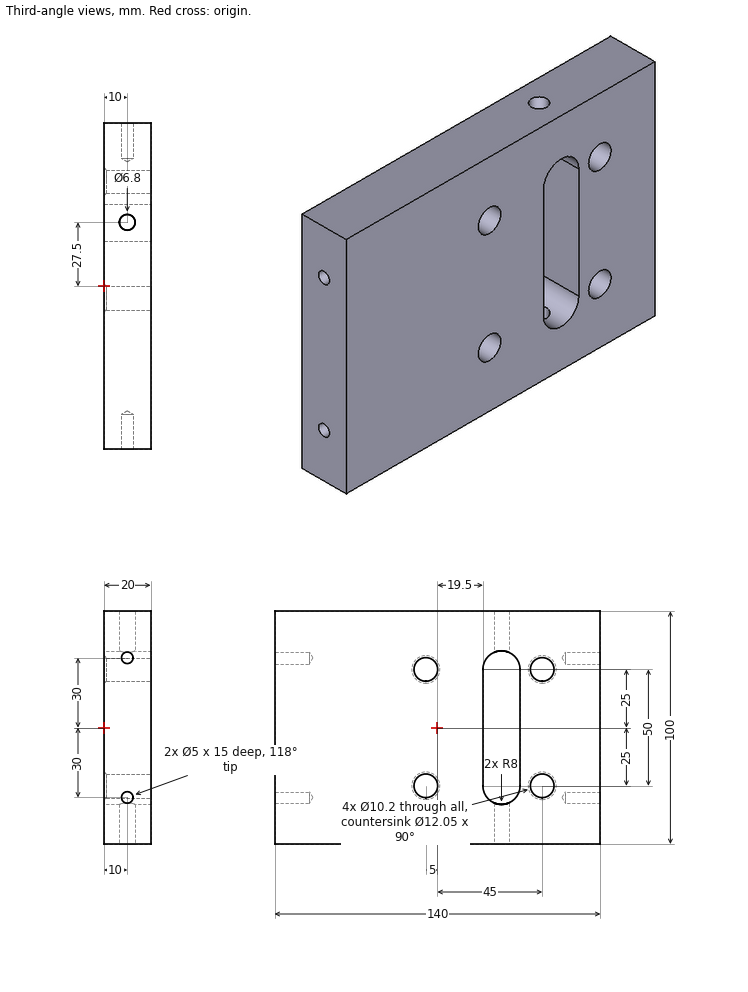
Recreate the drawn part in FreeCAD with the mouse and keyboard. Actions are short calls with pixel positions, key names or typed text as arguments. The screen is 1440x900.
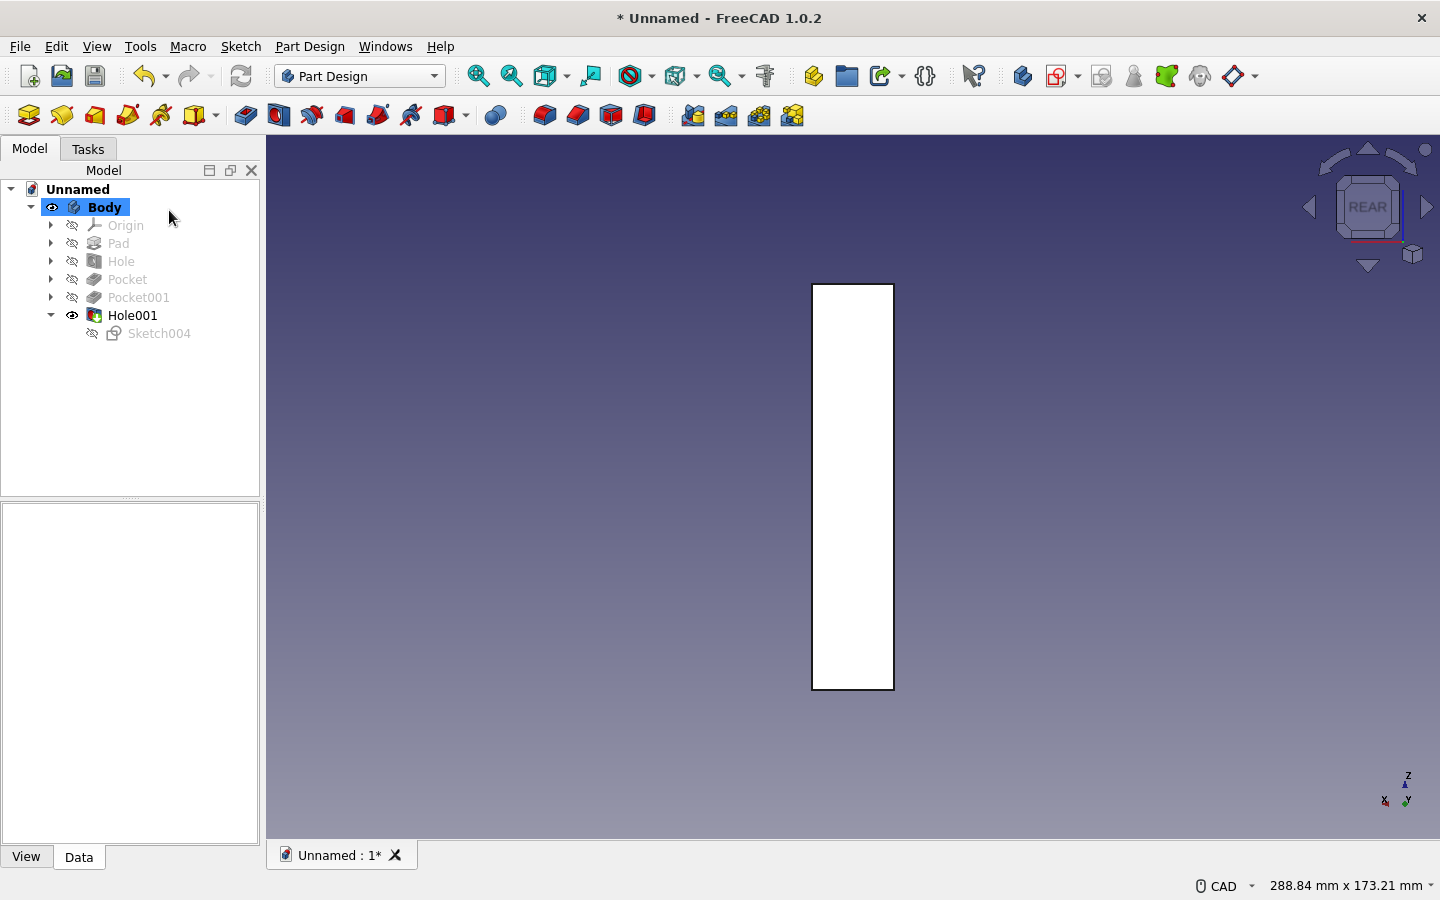
click(853, 486)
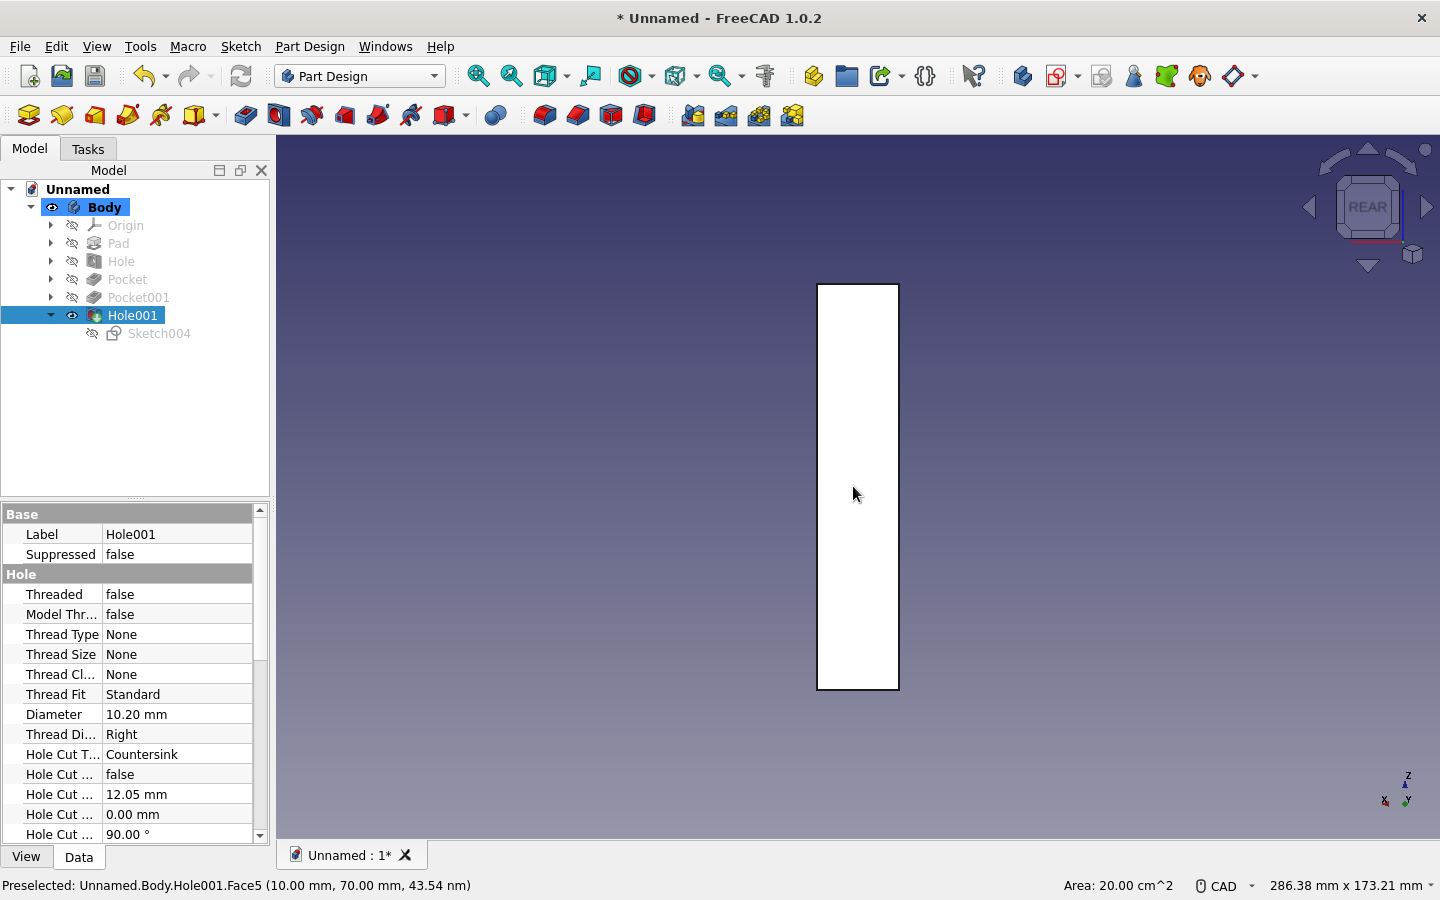
click(1056, 76)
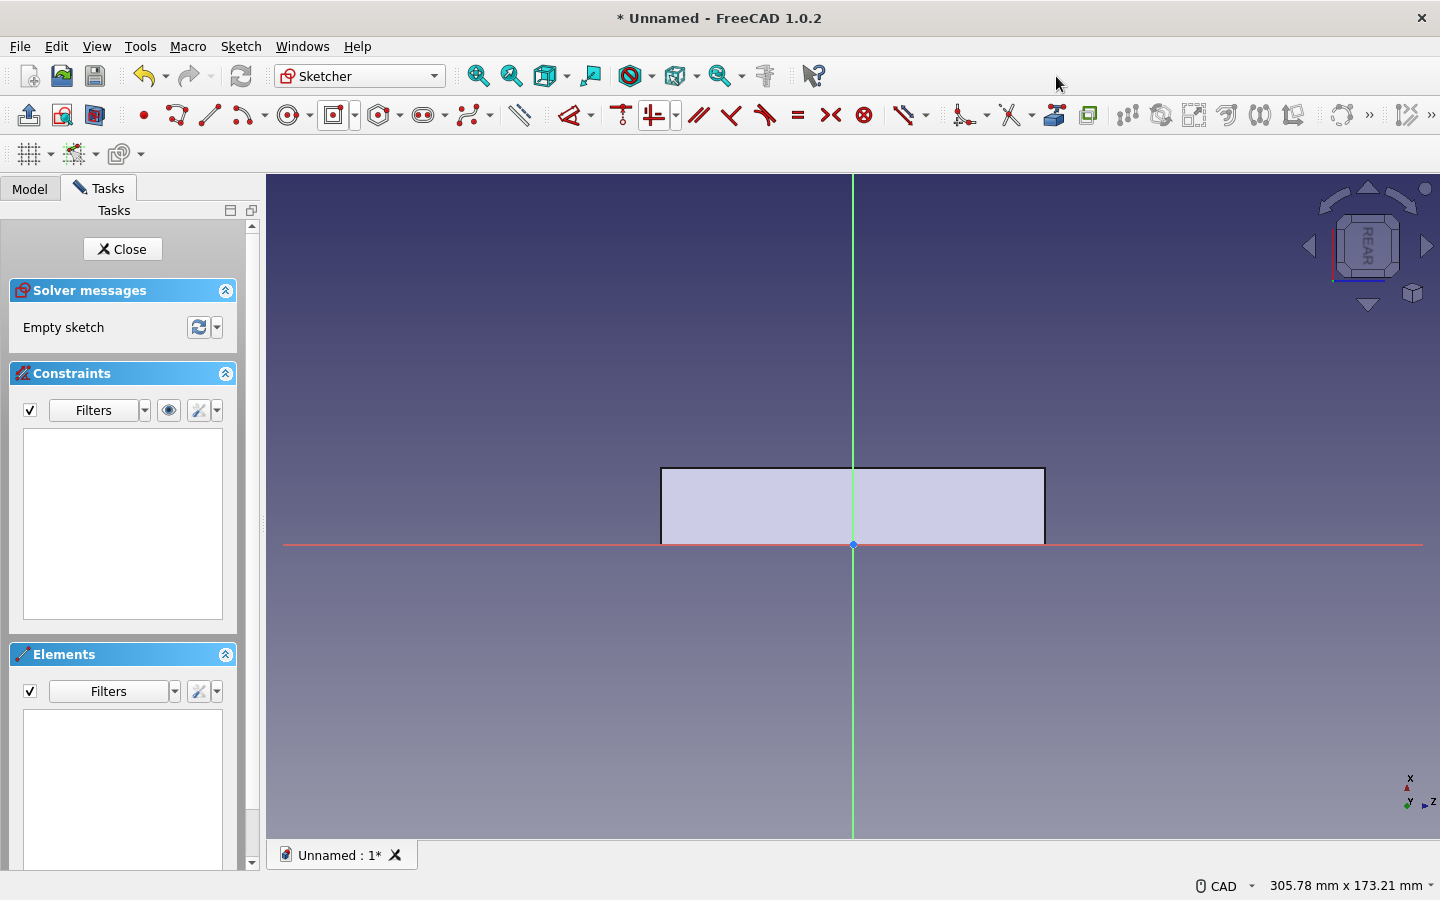
scroll(893, 529, up, 5)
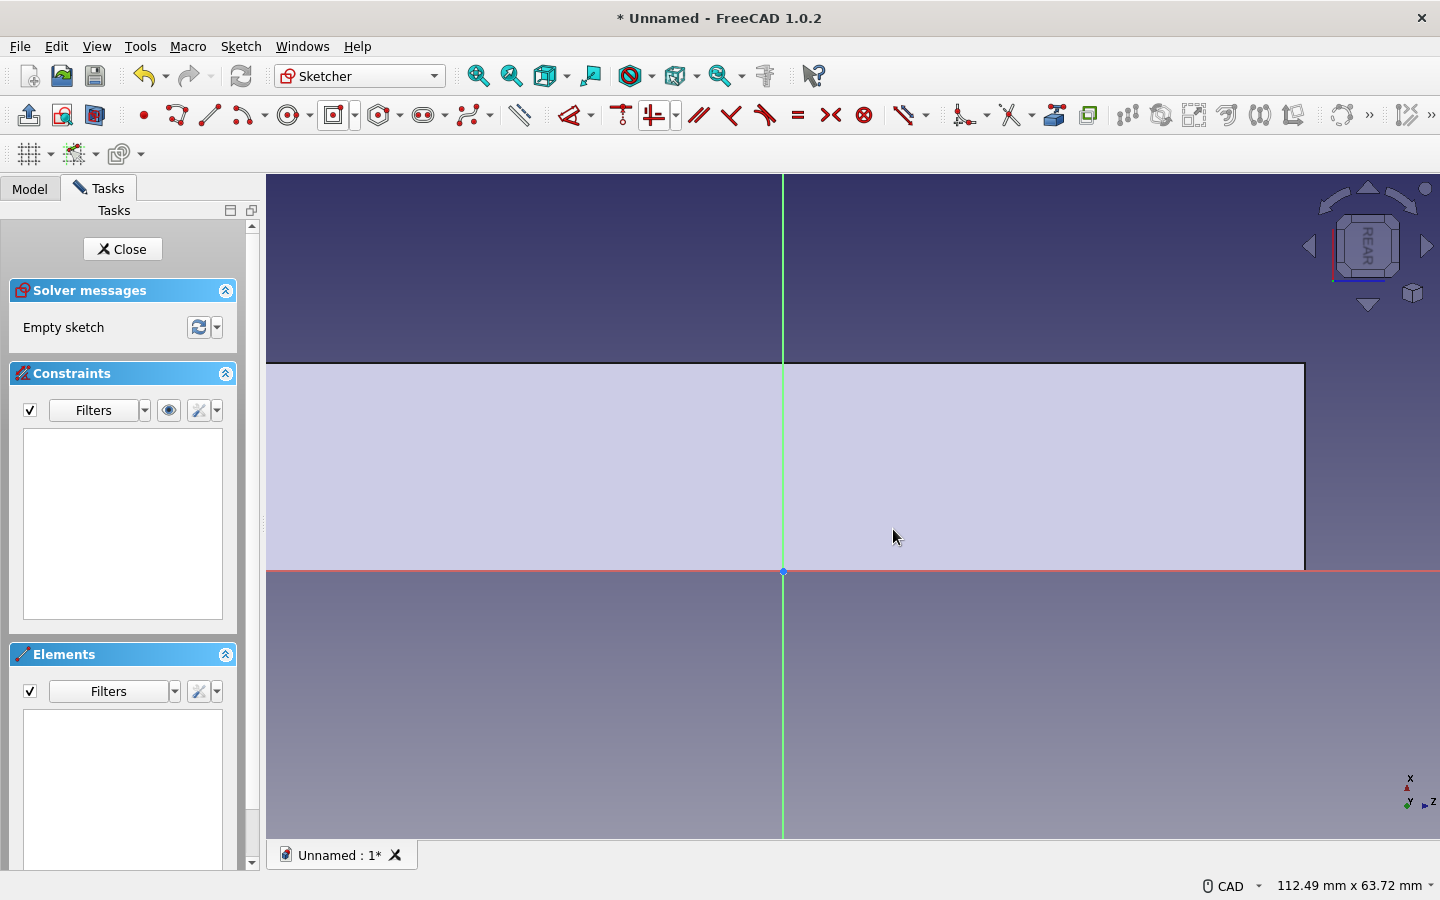
click(288, 116)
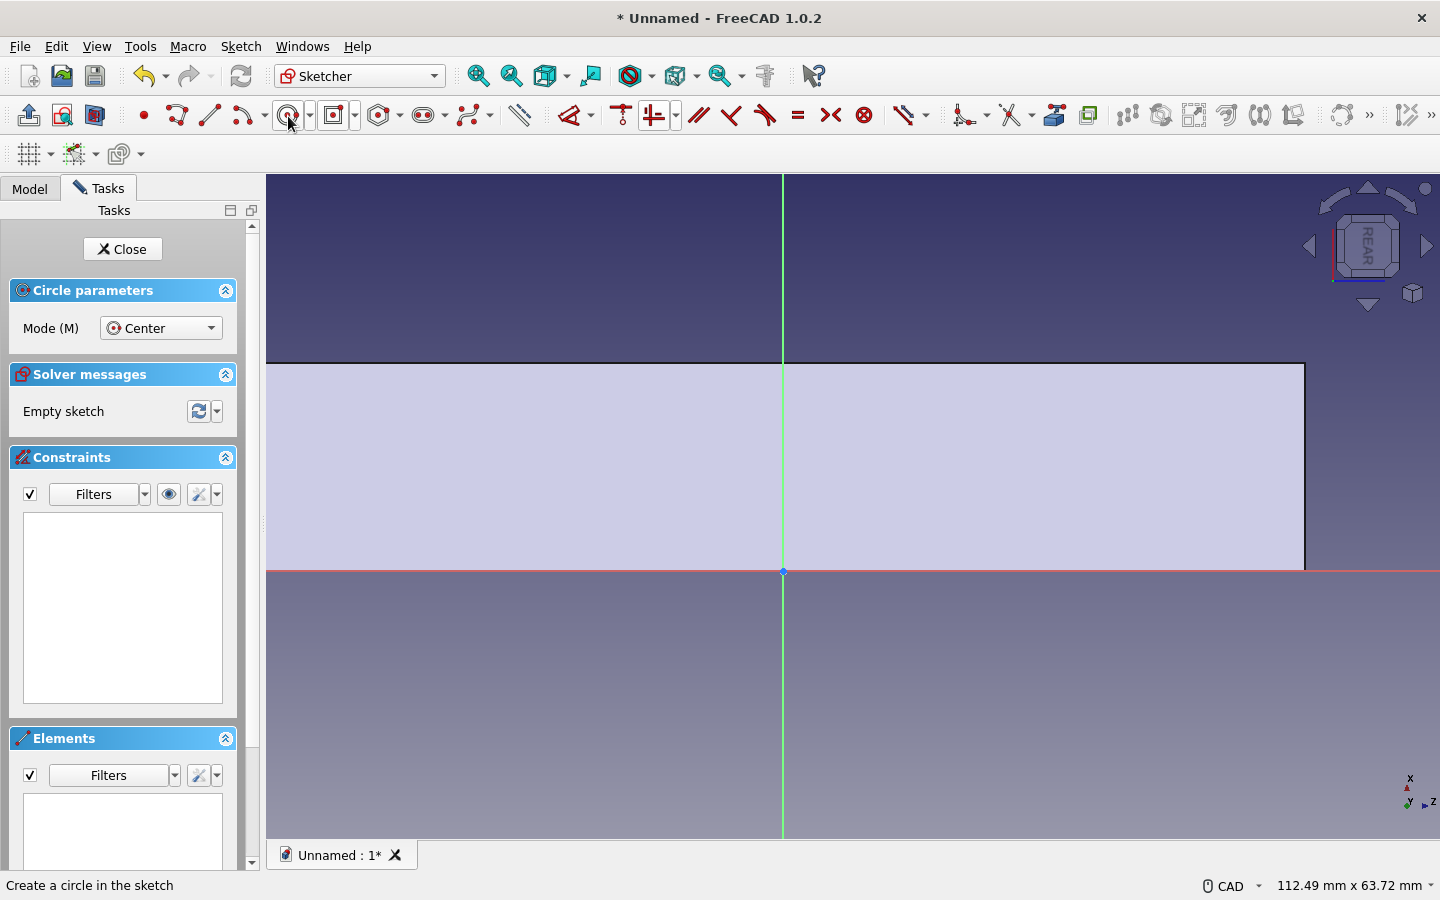
click(470, 467)
move(489, 448)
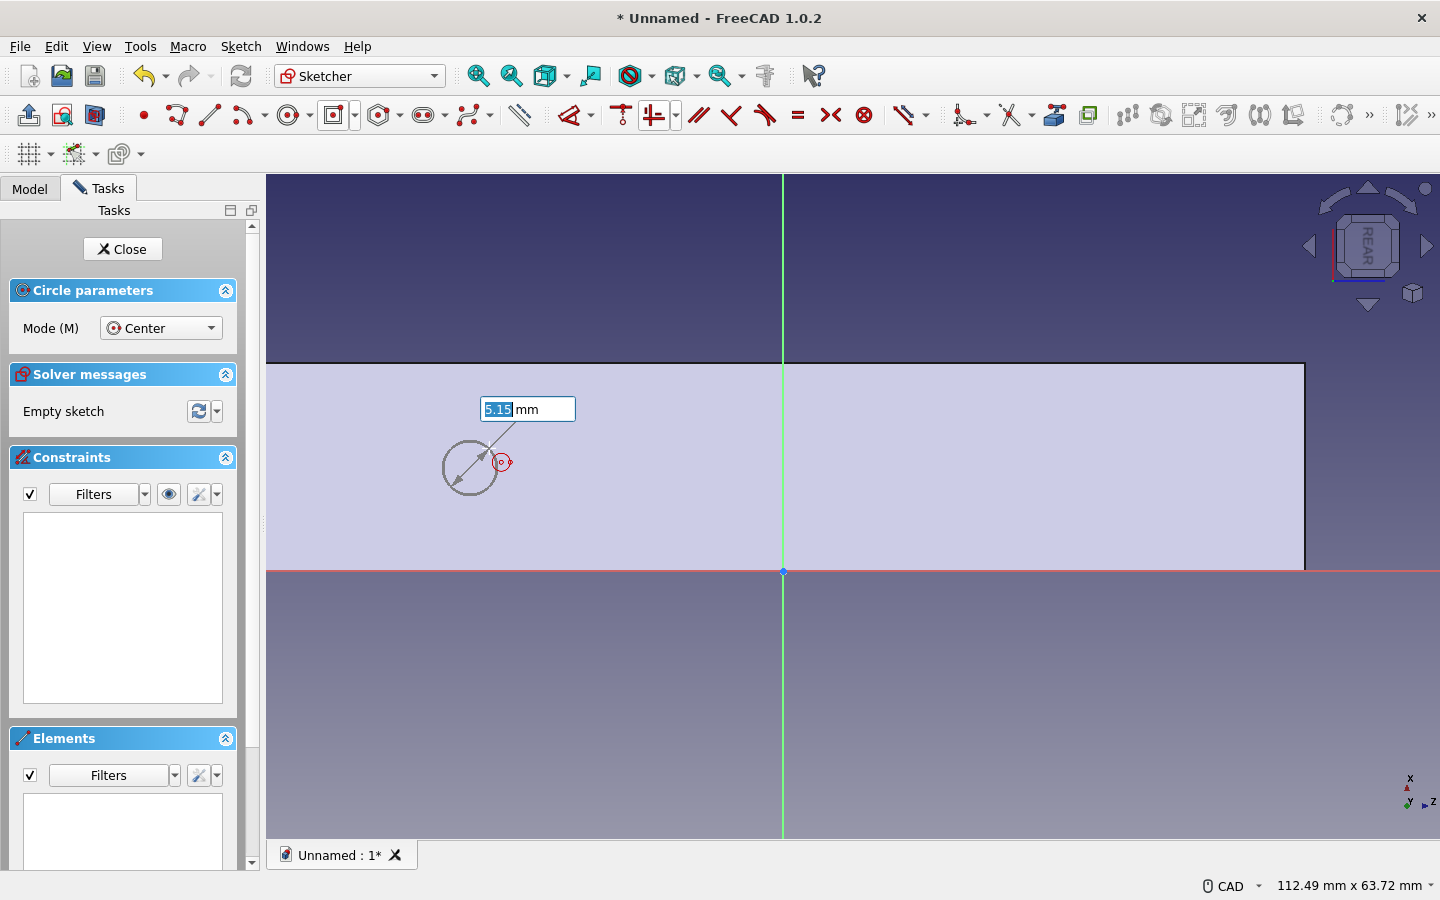
text(5)
key(Return)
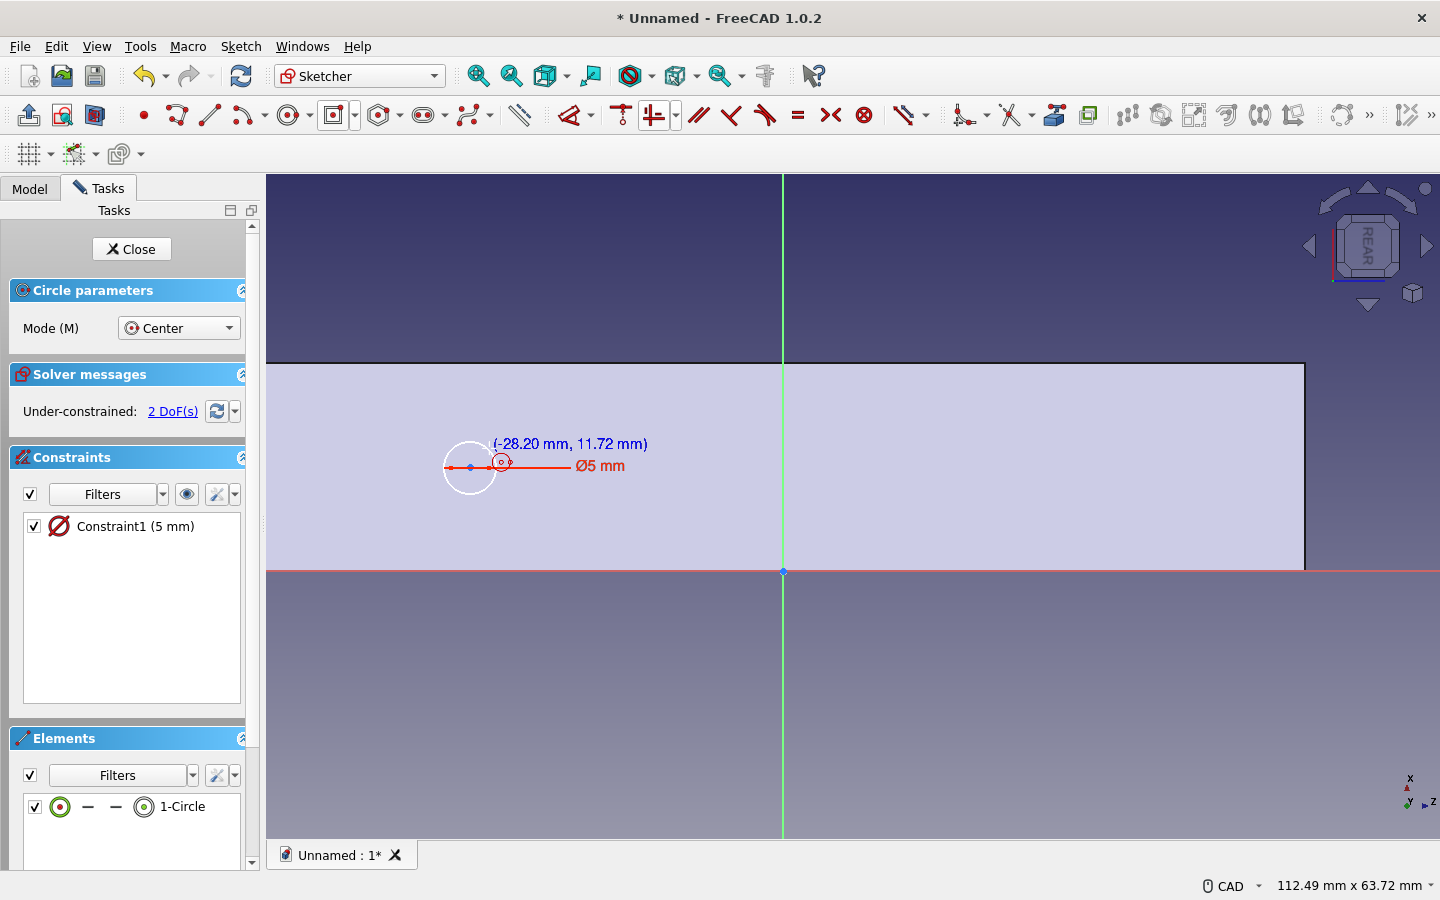
click(1096, 467)
move(1115, 448)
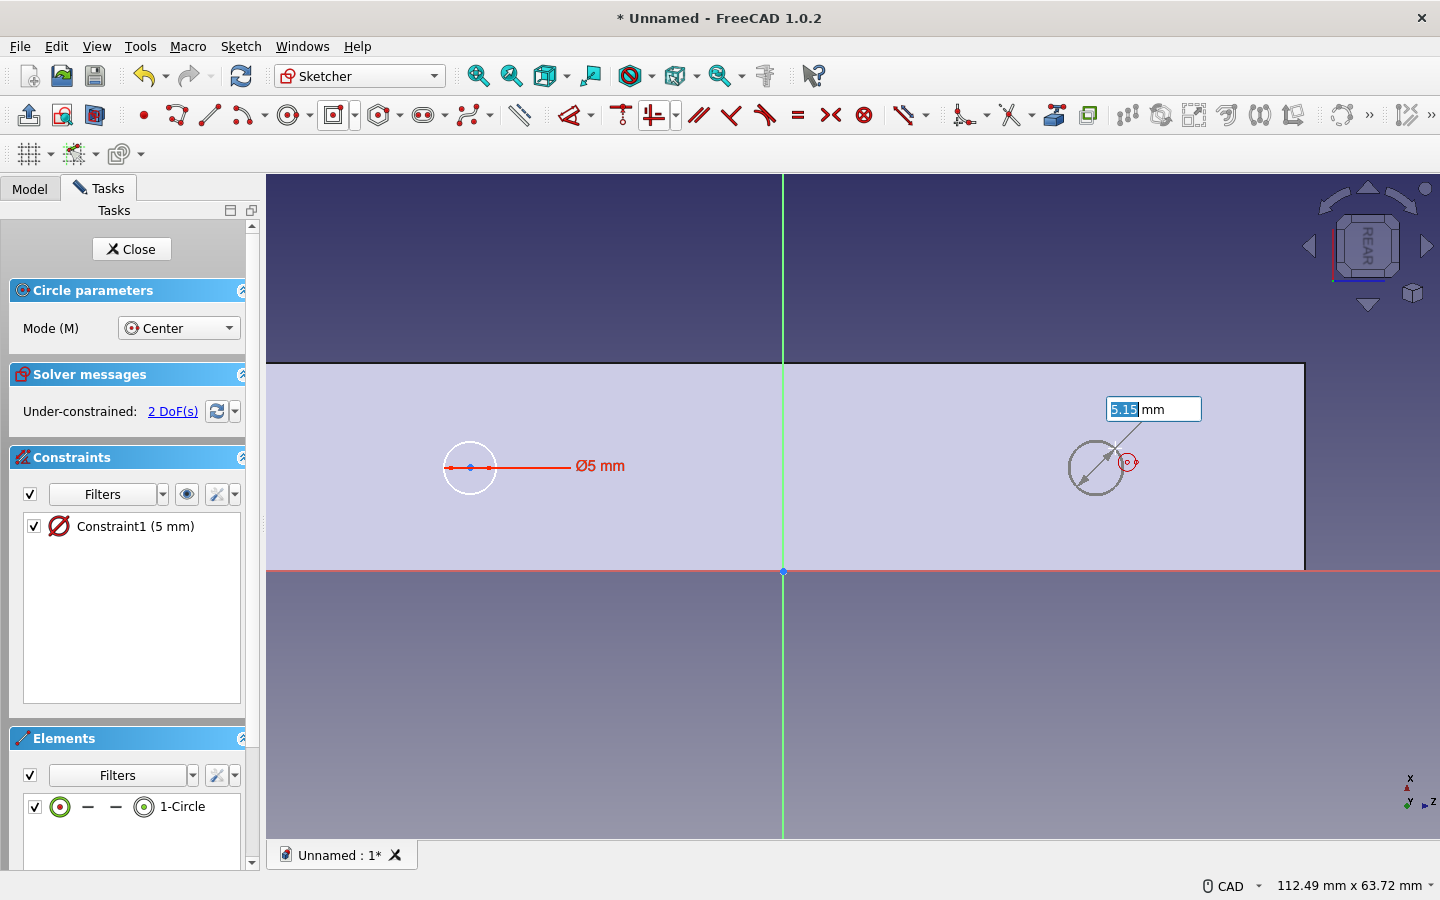
text(5)
key(Return)
key(Escape)